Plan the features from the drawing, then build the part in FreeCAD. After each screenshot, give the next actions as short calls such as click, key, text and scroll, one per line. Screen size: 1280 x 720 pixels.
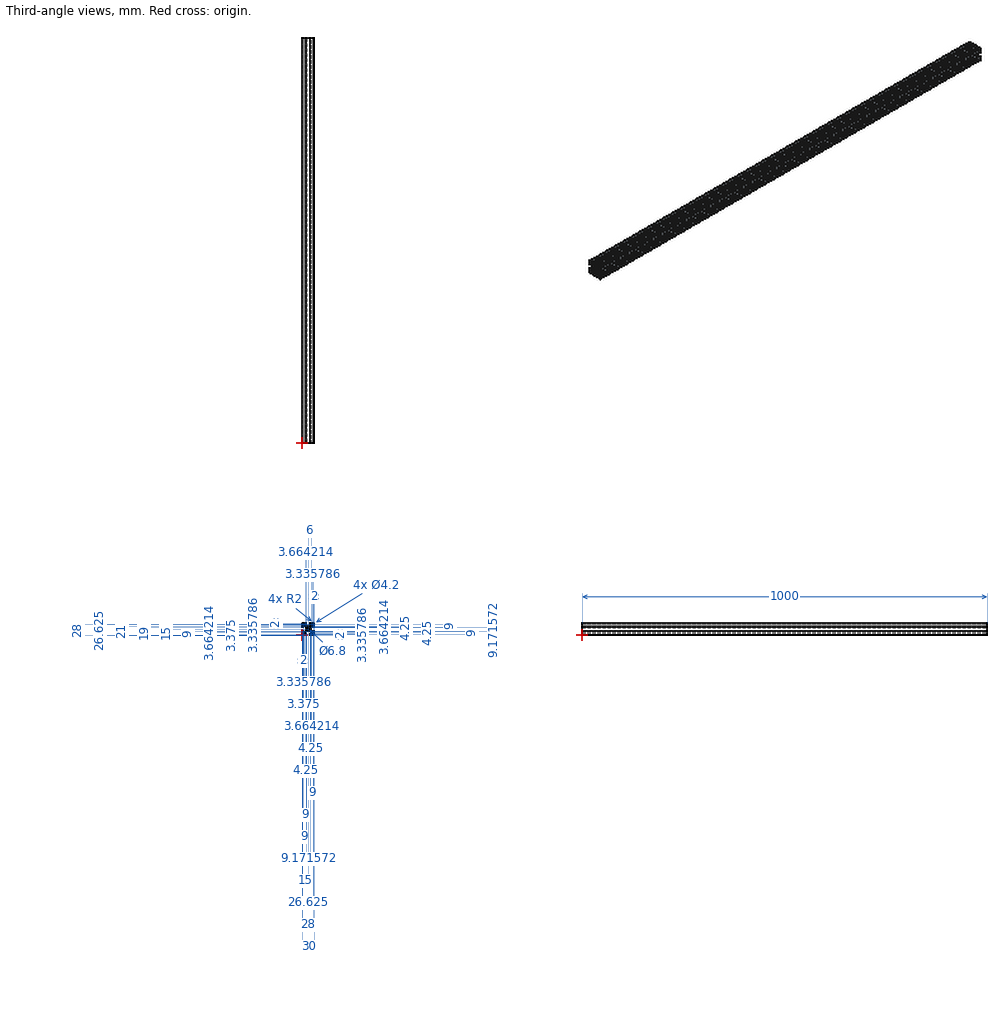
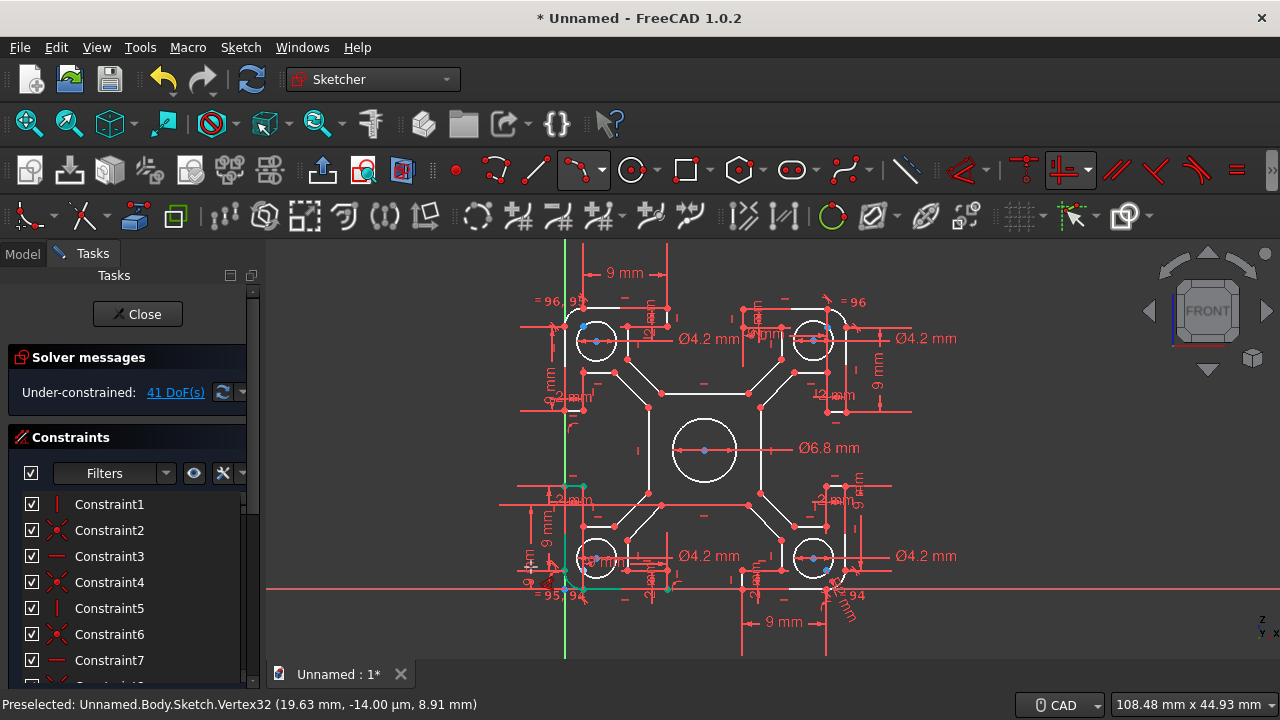
click(649, 493)
click(607, 623)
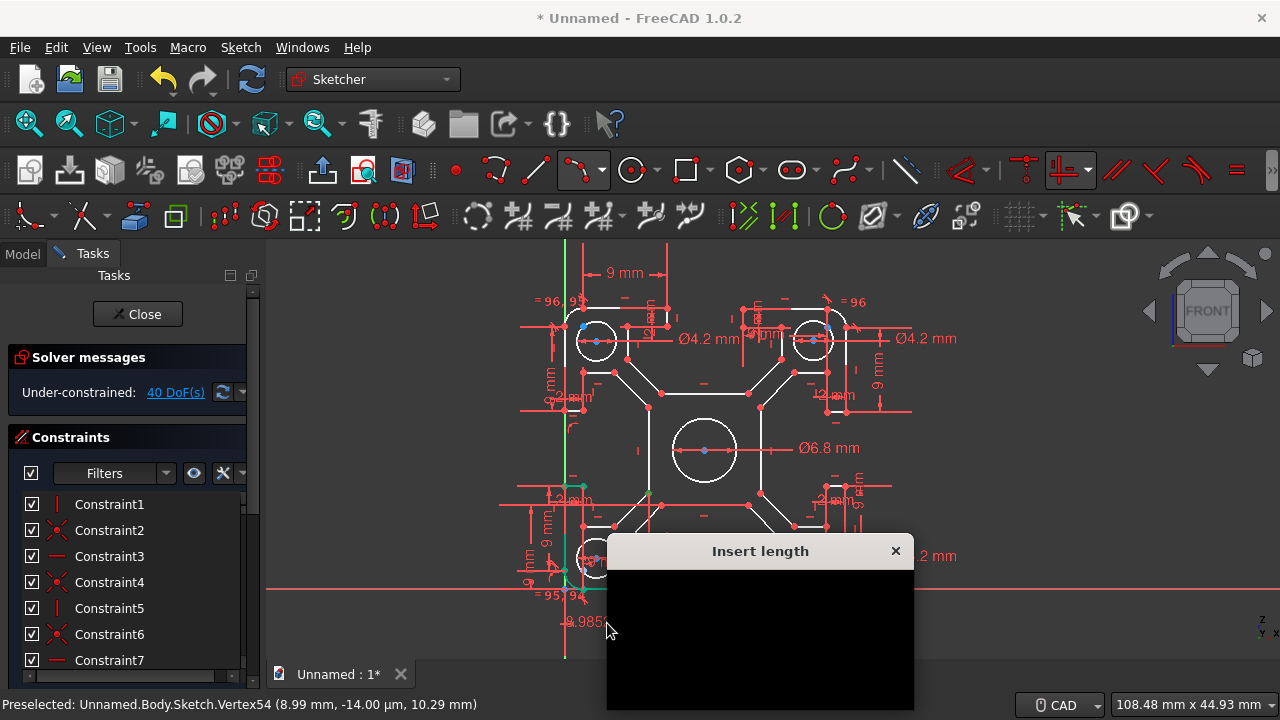
text(9)
key(Return)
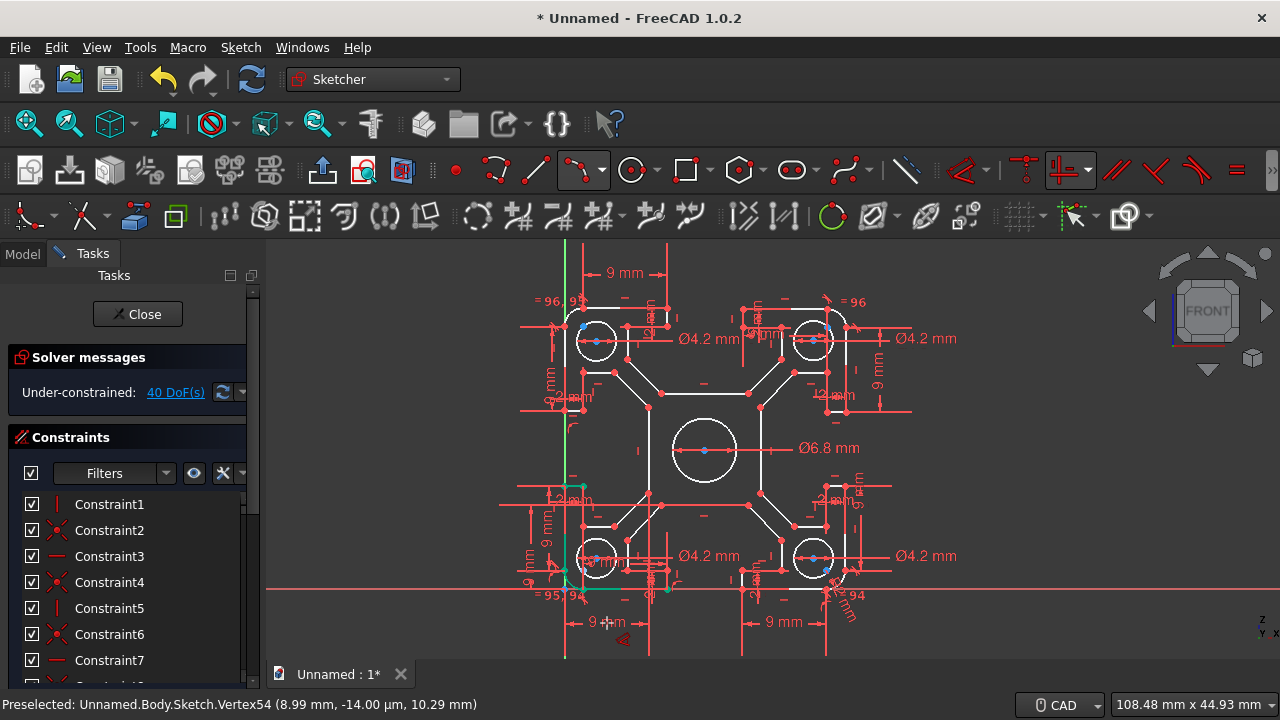
click(705, 450)
click(684, 623)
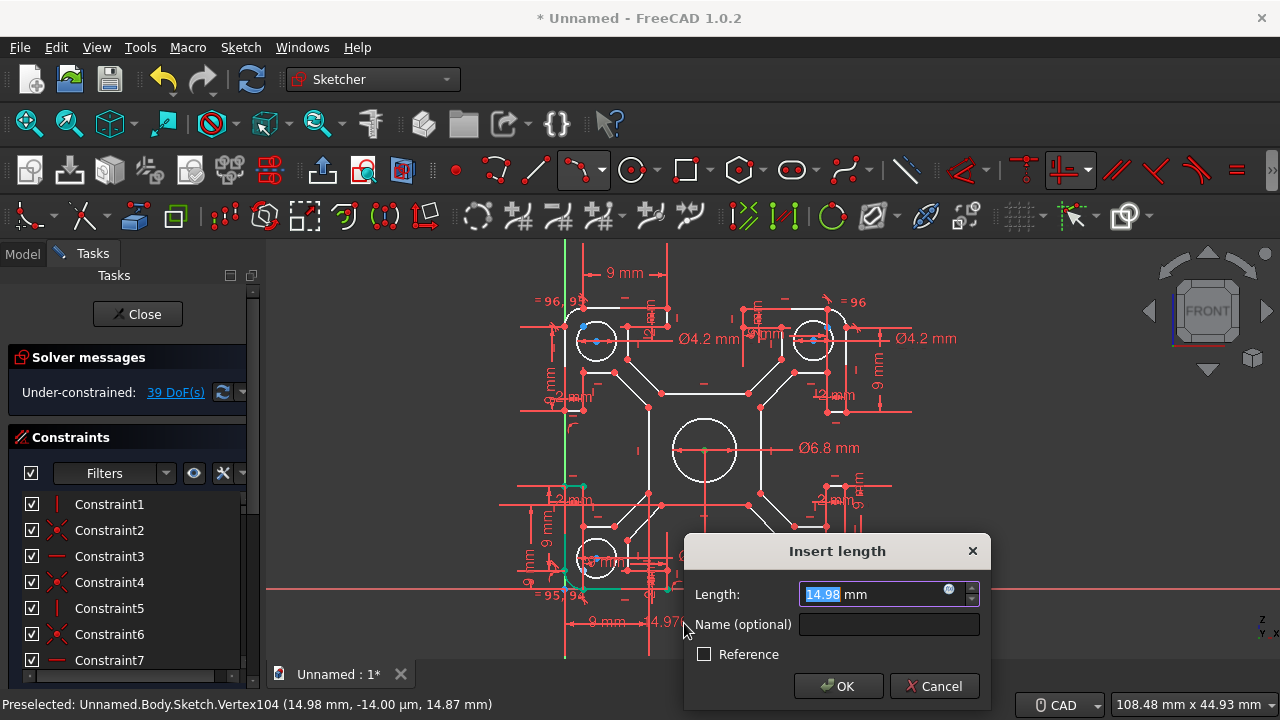
text(15)
key(Return)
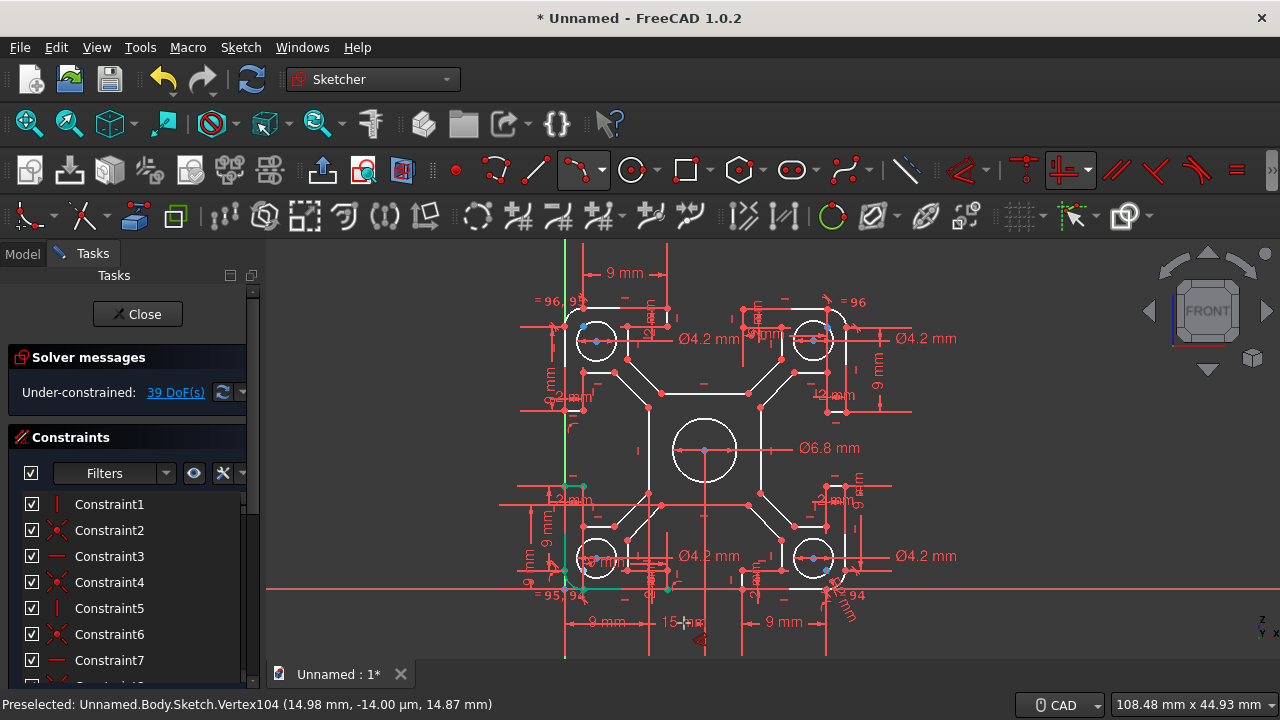
click(705, 450)
click(531, 471)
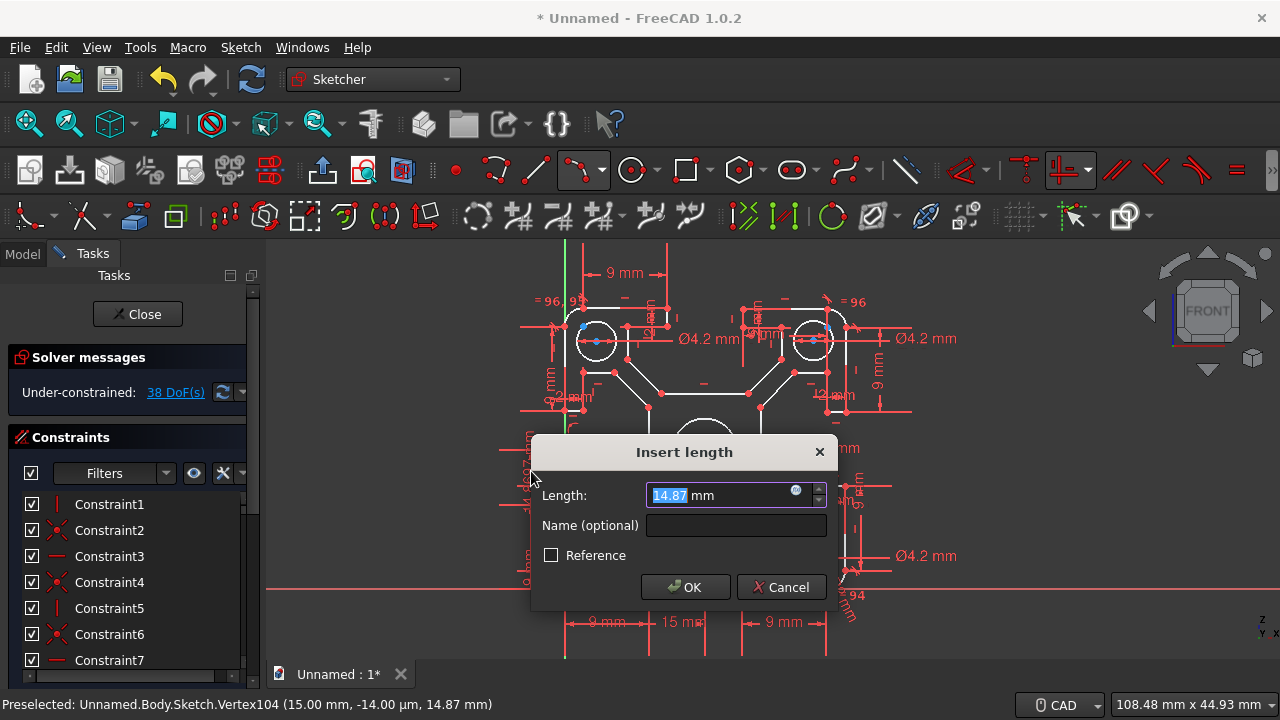
text(15)
key(Return)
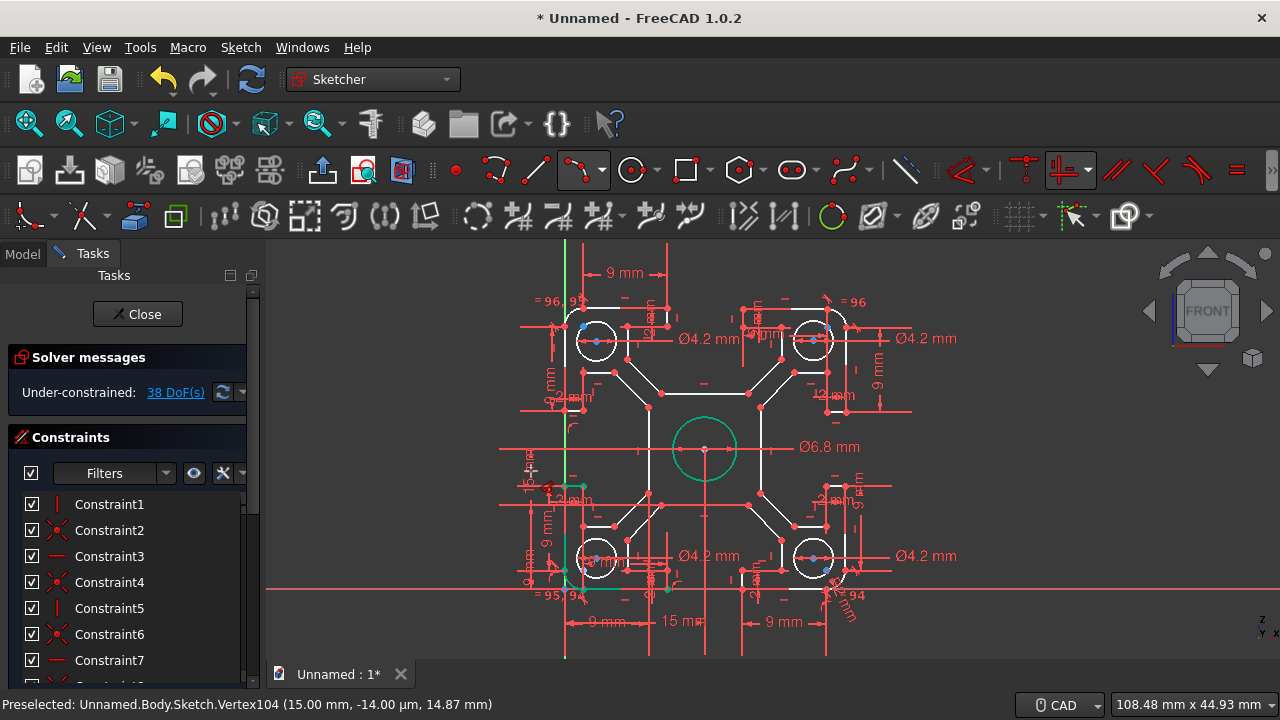
click(761, 407)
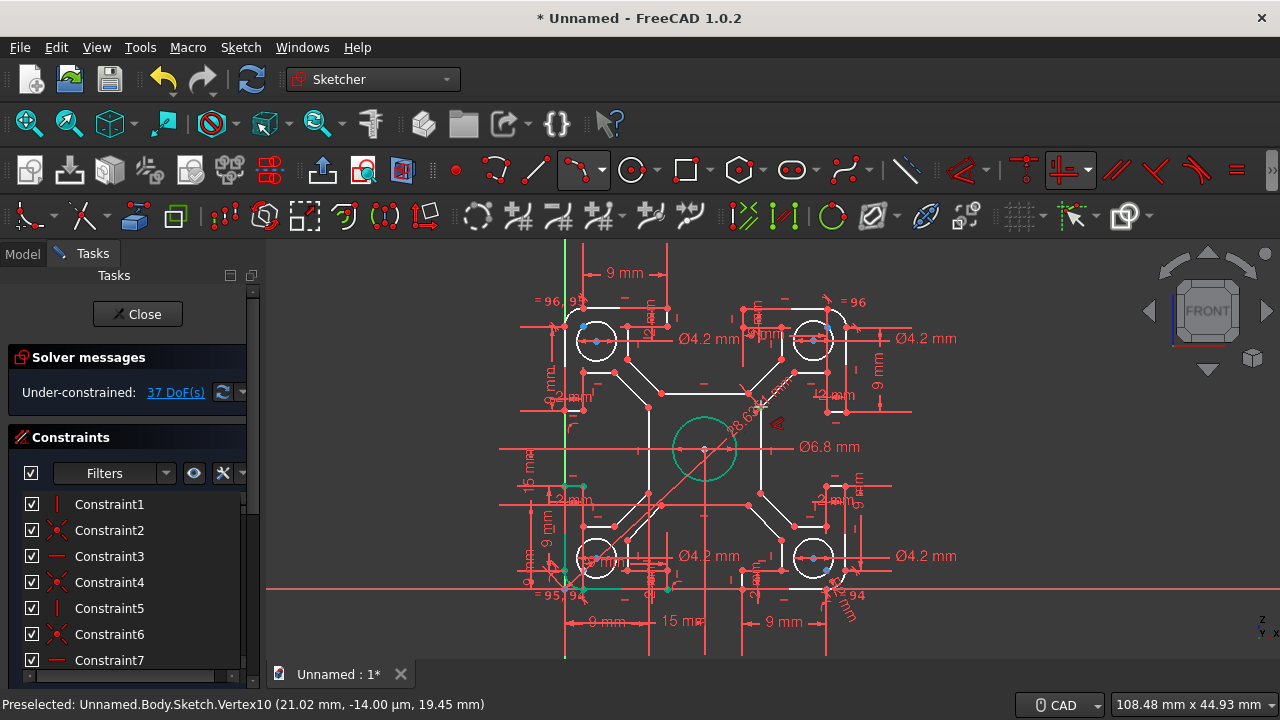
click(705, 449)
click(733, 373)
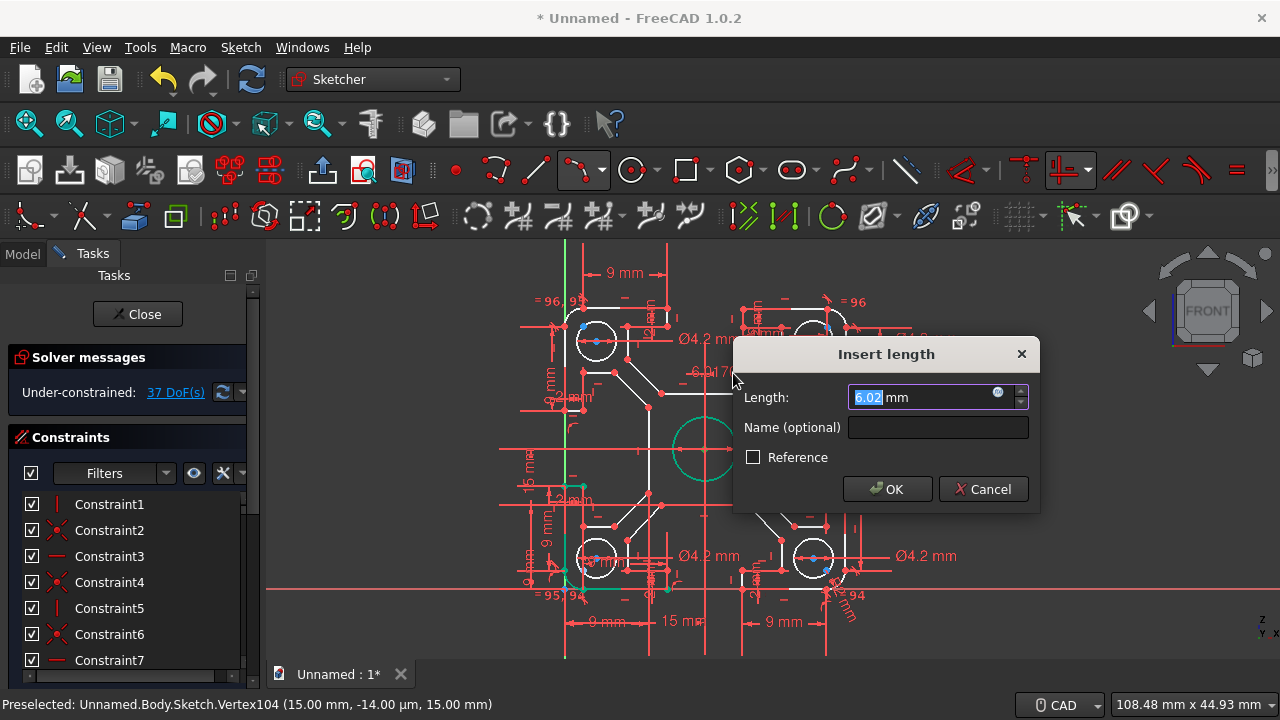
text(6)
key(Return)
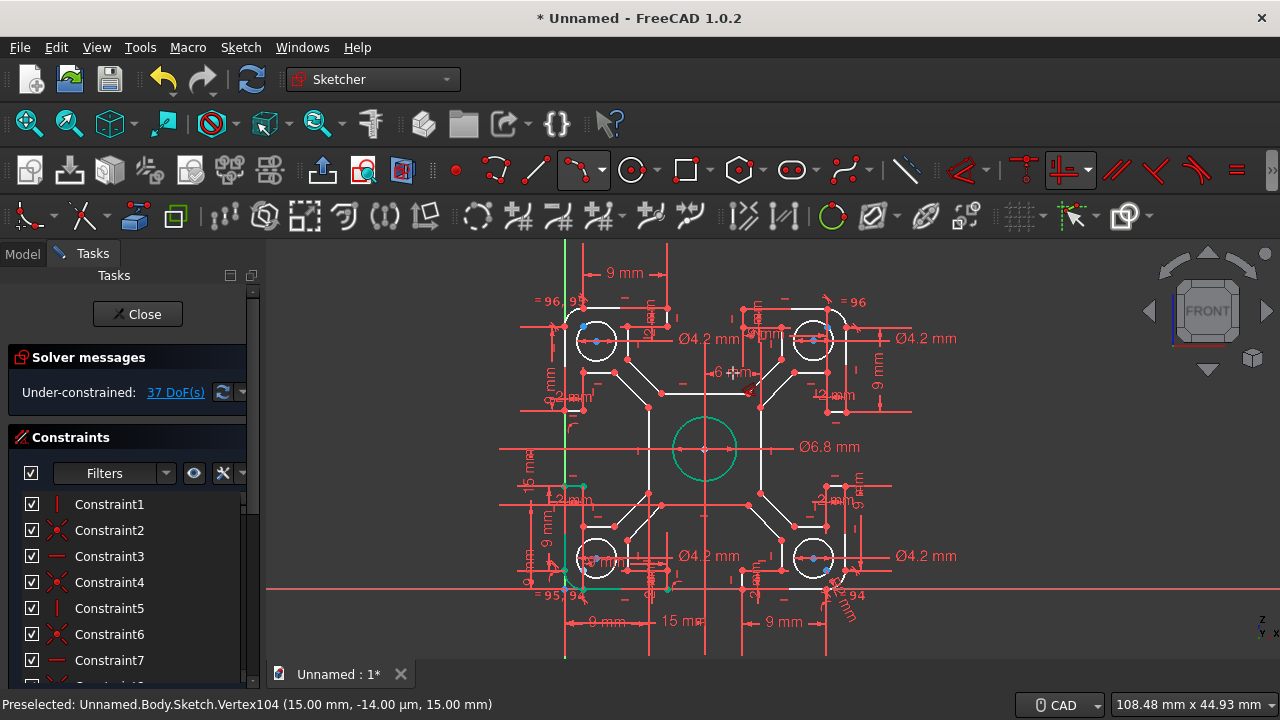
click(846, 328)
click(705, 294)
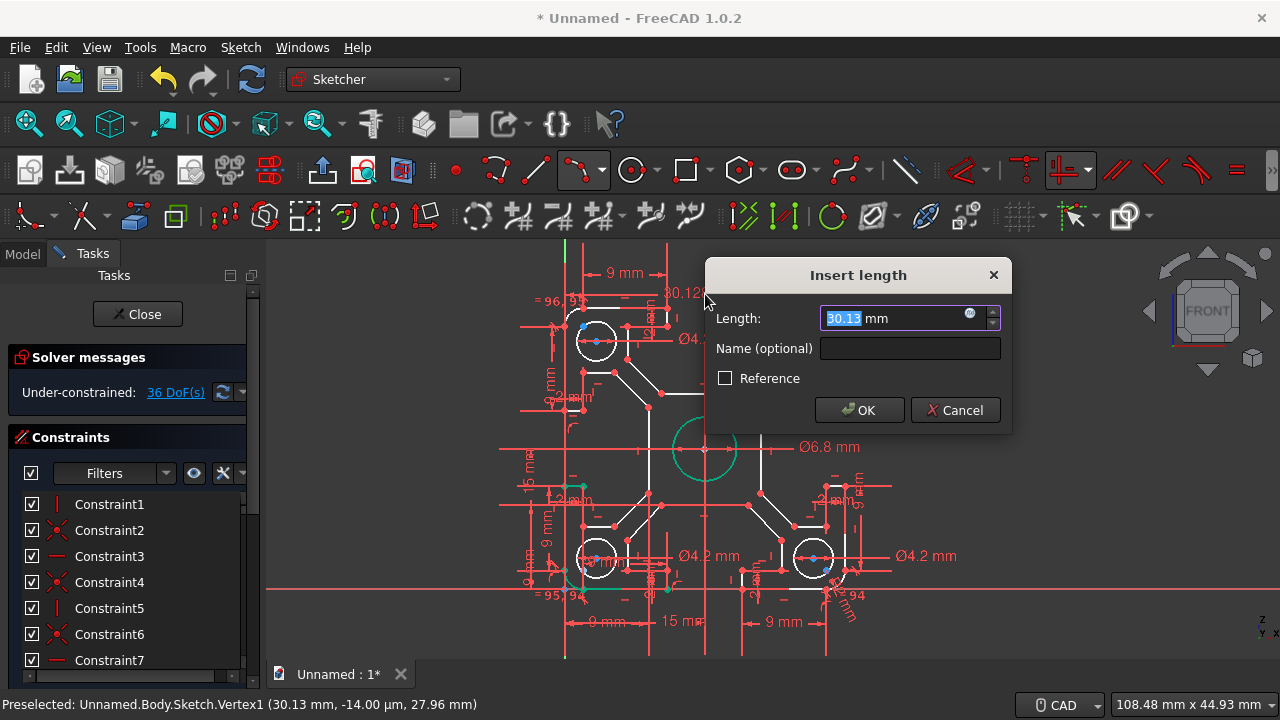
text(30)
key(Return)